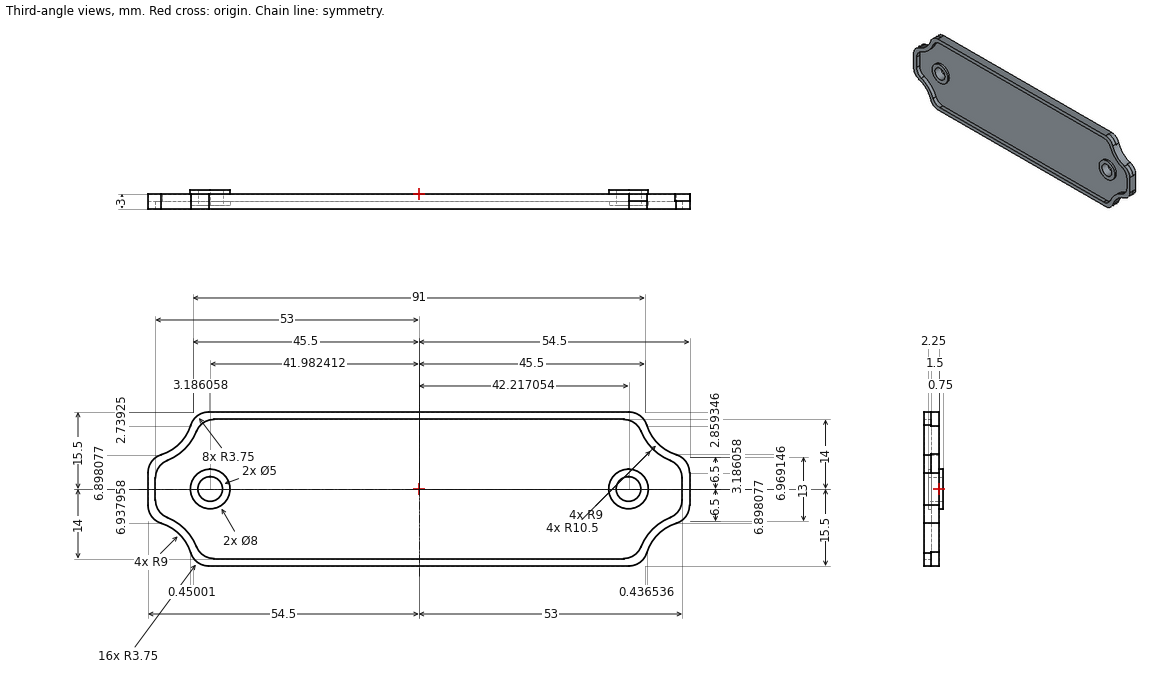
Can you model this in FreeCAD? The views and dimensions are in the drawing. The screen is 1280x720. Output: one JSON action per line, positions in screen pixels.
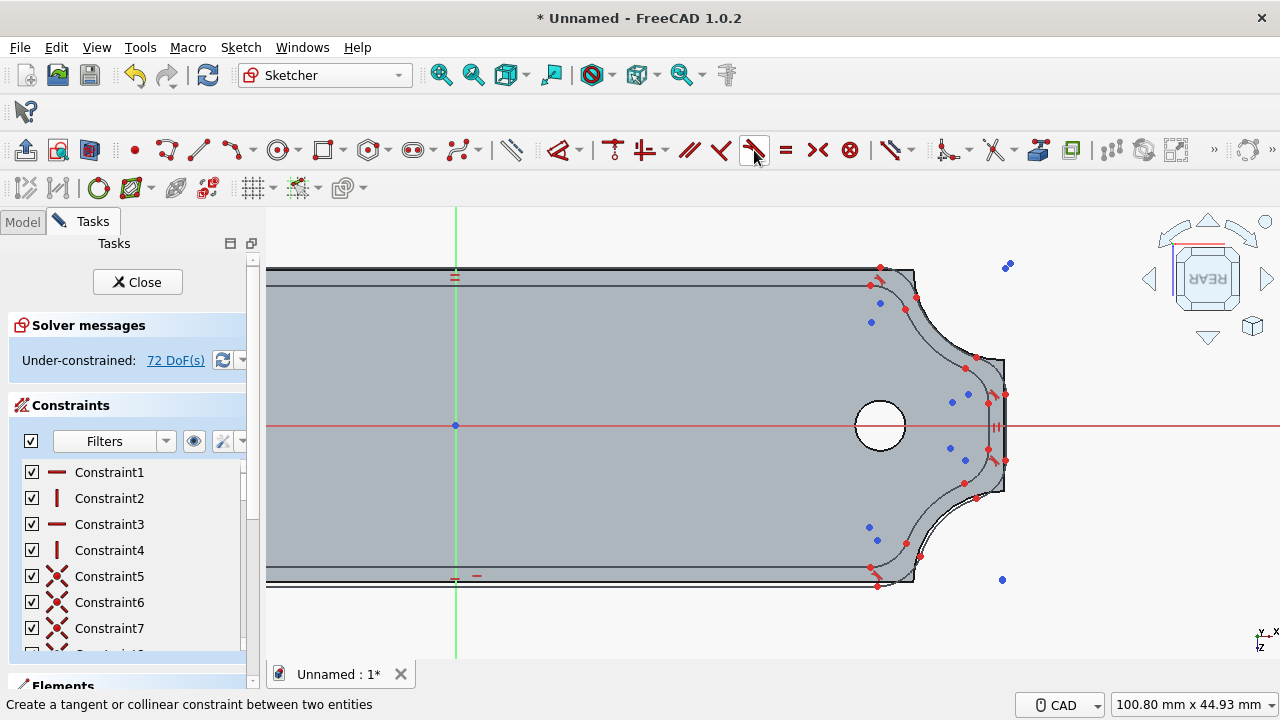
{"action": "scroll", "coordinate": [1007, 442], "scroll_direction": "down", "scroll_amount": 3}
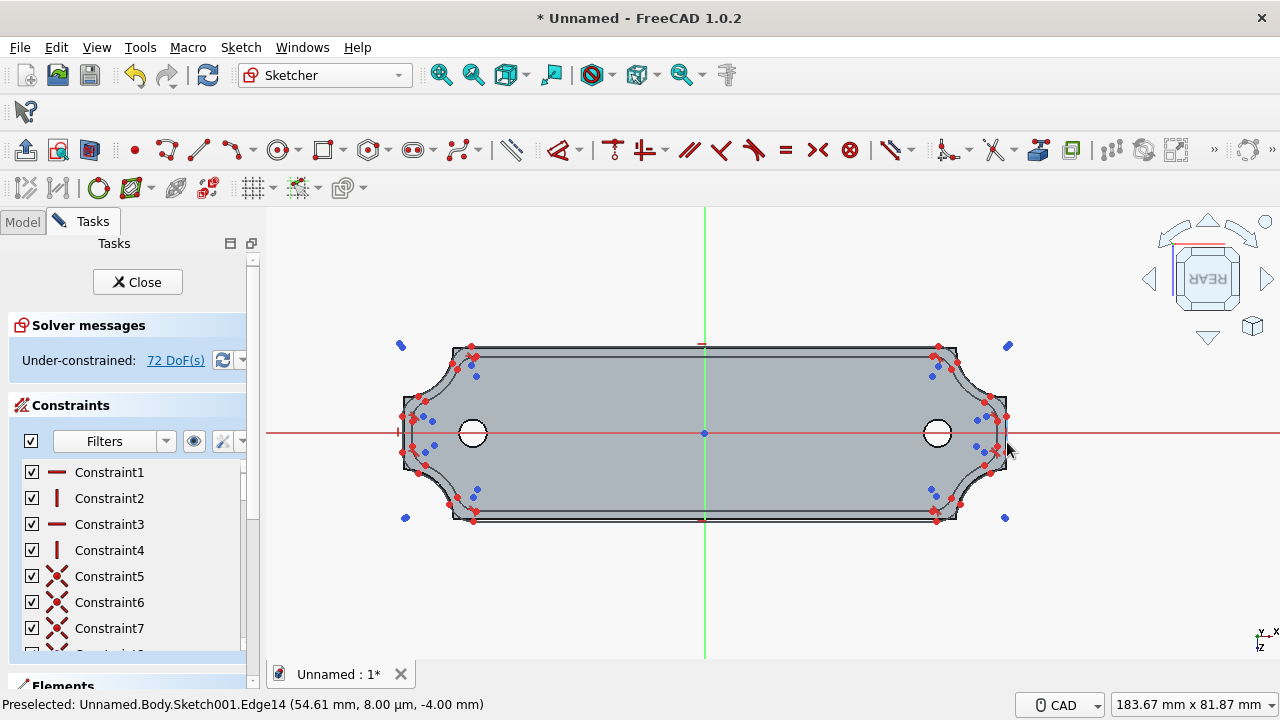
{"action": "scroll", "coordinate": [463, 348], "scroll_direction": "up", "scroll_amount": 3}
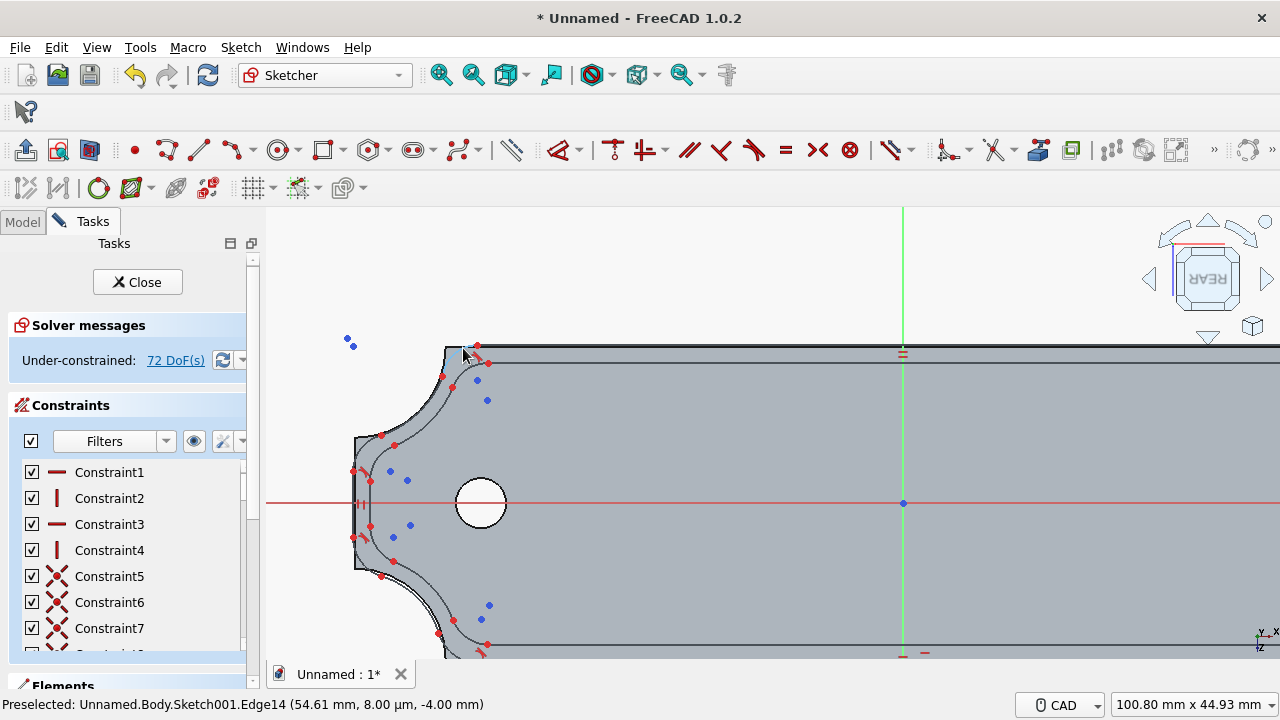
{"action": "left_click", "coordinate": [463, 348]}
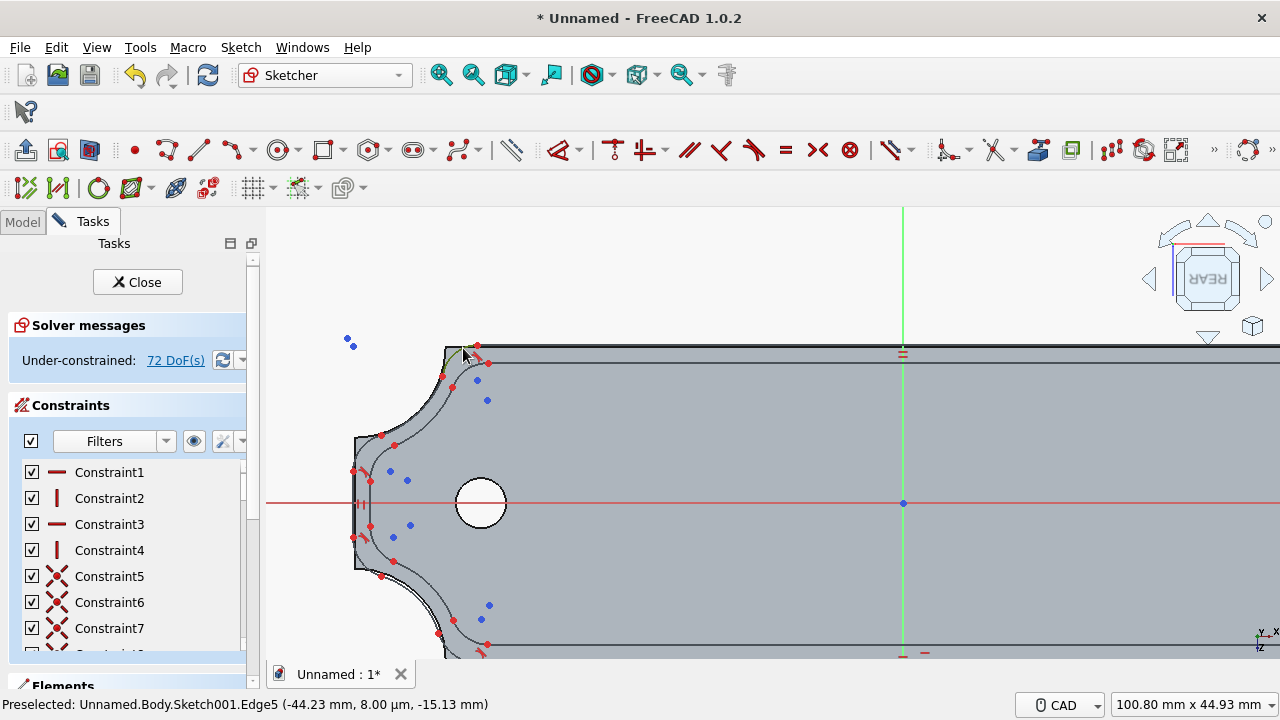
{"action": "left_click", "coordinate": [405, 423]}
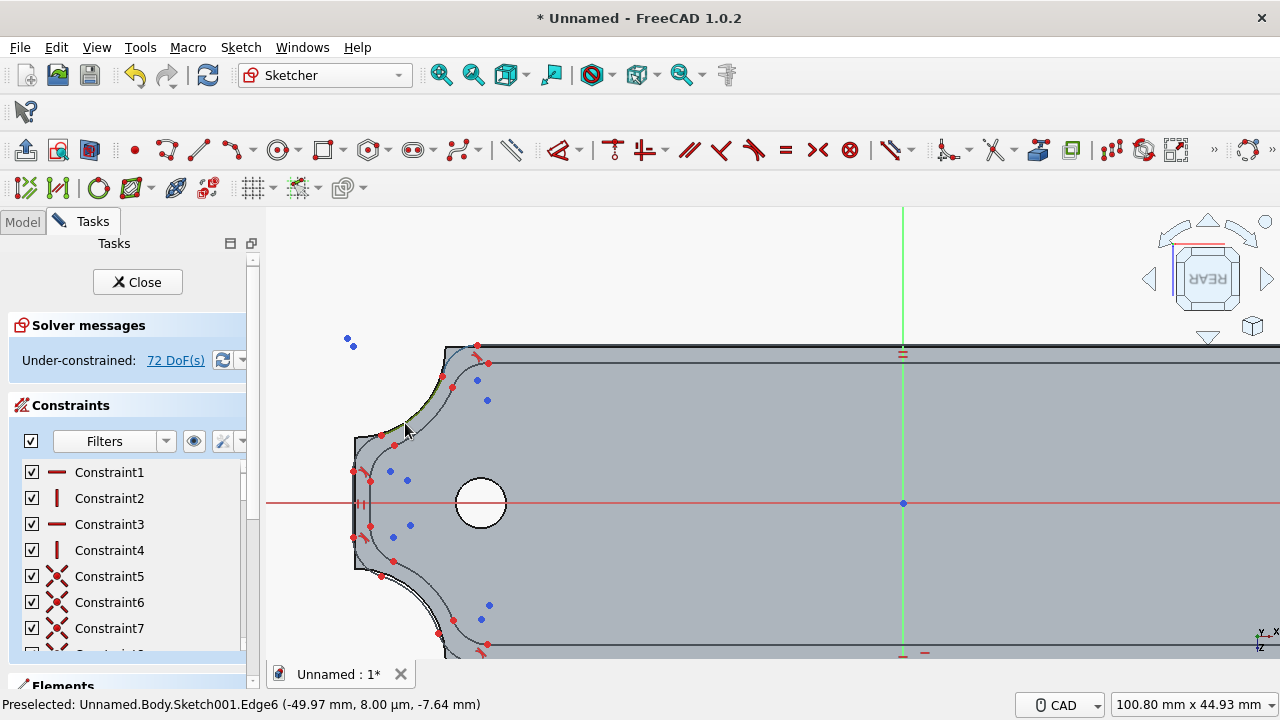
{"action": "left_click", "coordinate": [754, 150]}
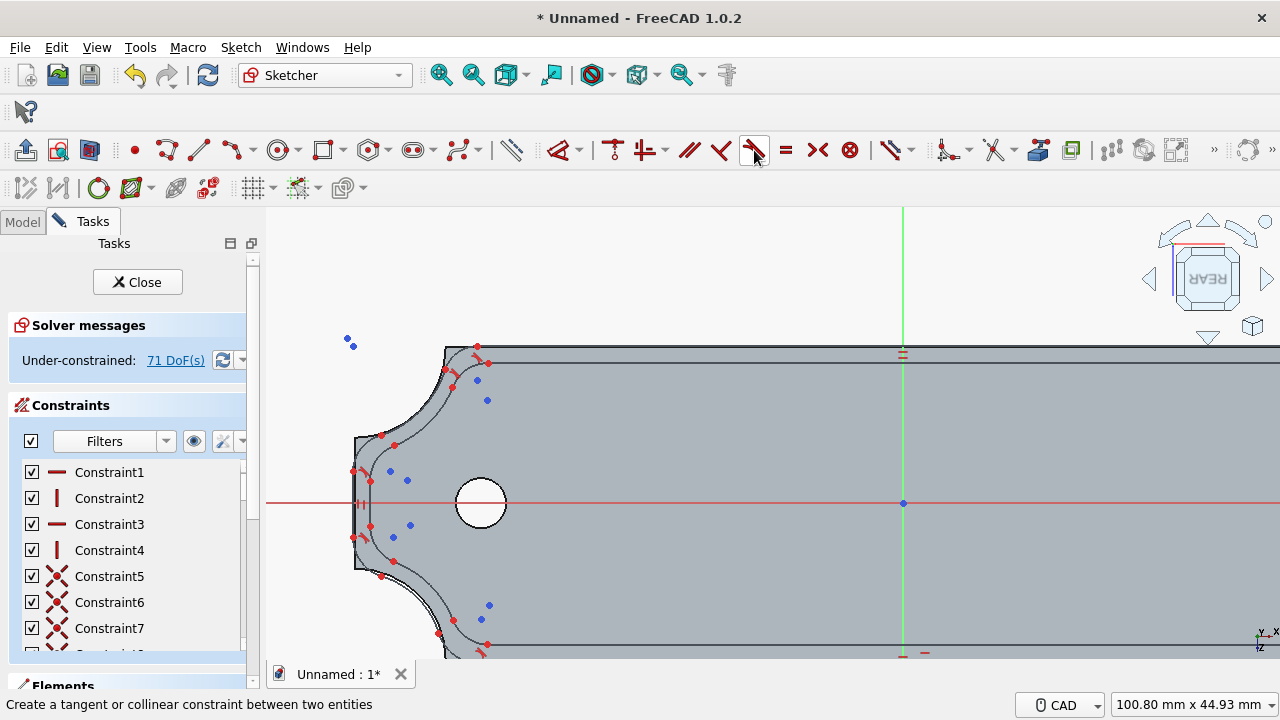
{"action": "left_click", "coordinate": [407, 422]}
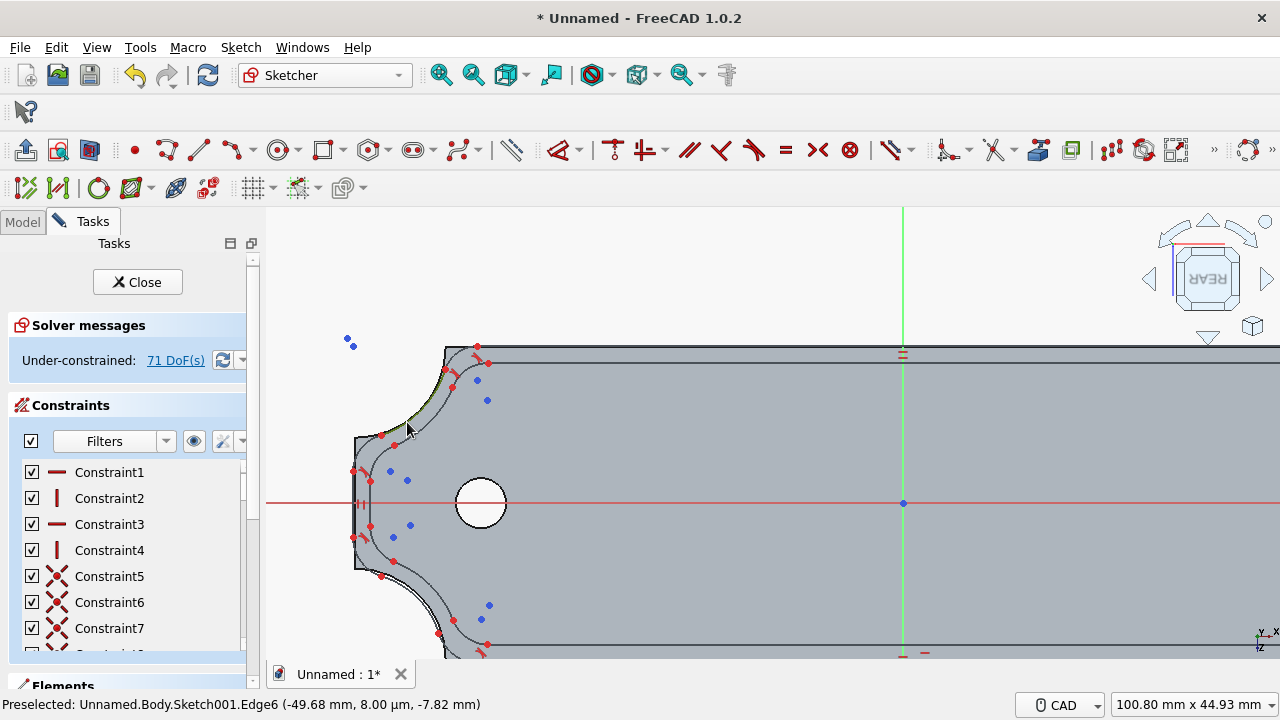
{"action": "left_click", "coordinate": [368, 442]}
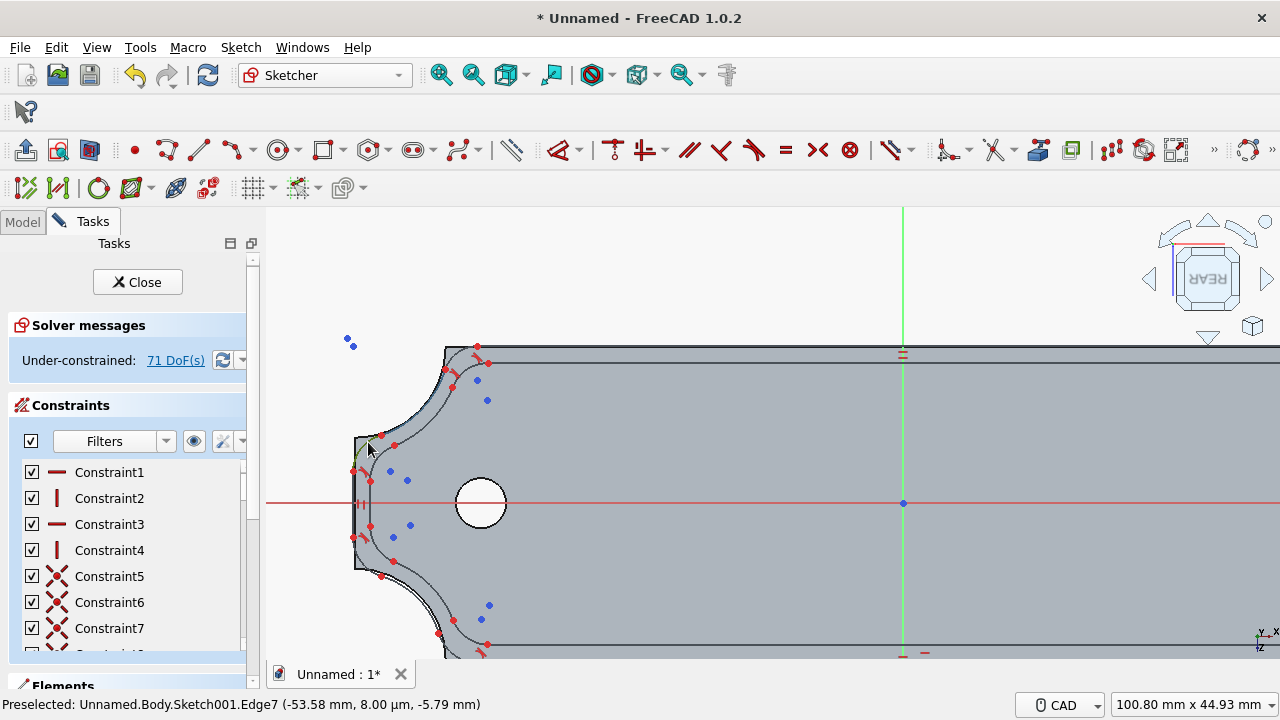
{"action": "left_click", "coordinate": [754, 150]}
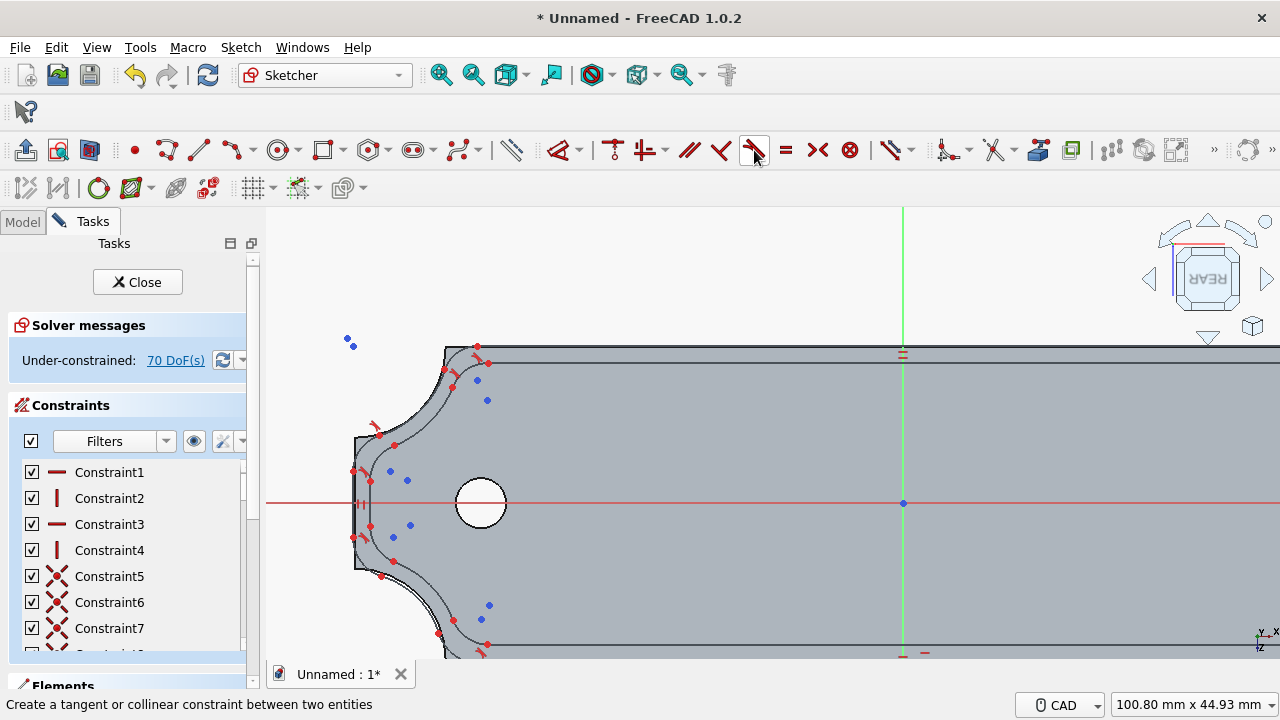
{"action": "left_click", "coordinate": [356, 553]}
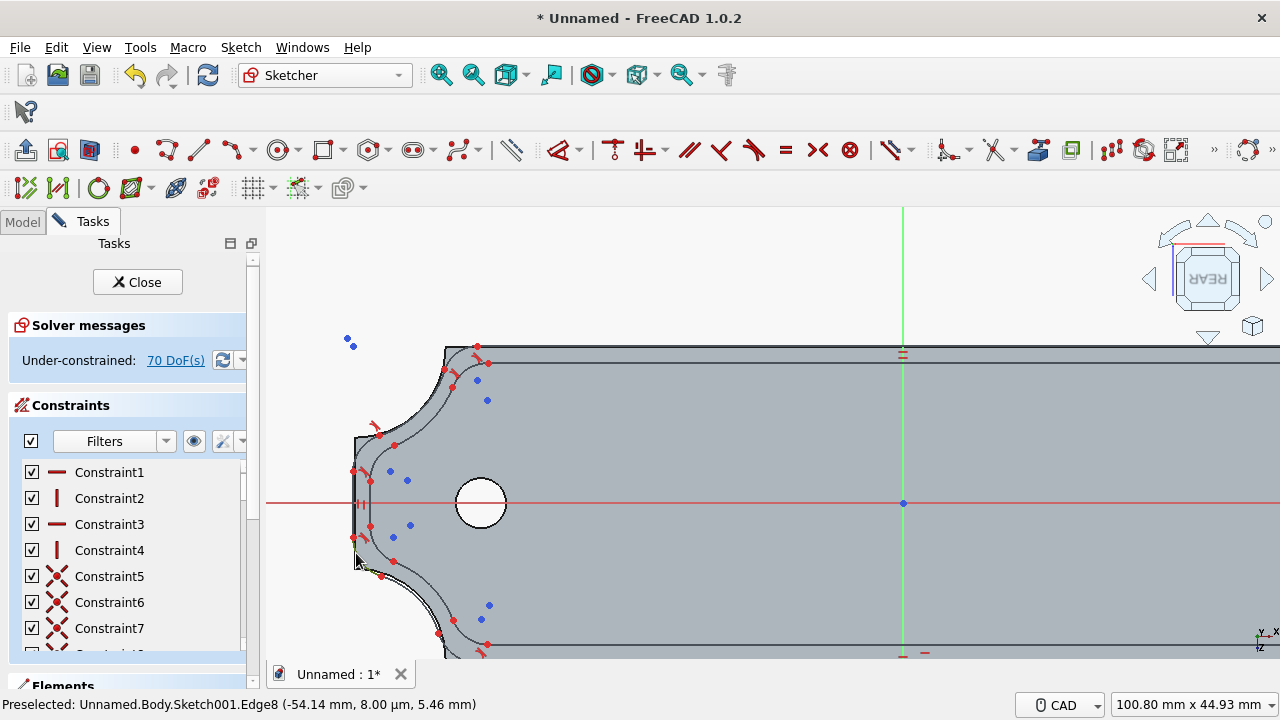
{"action": "left_click", "coordinate": [428, 611]}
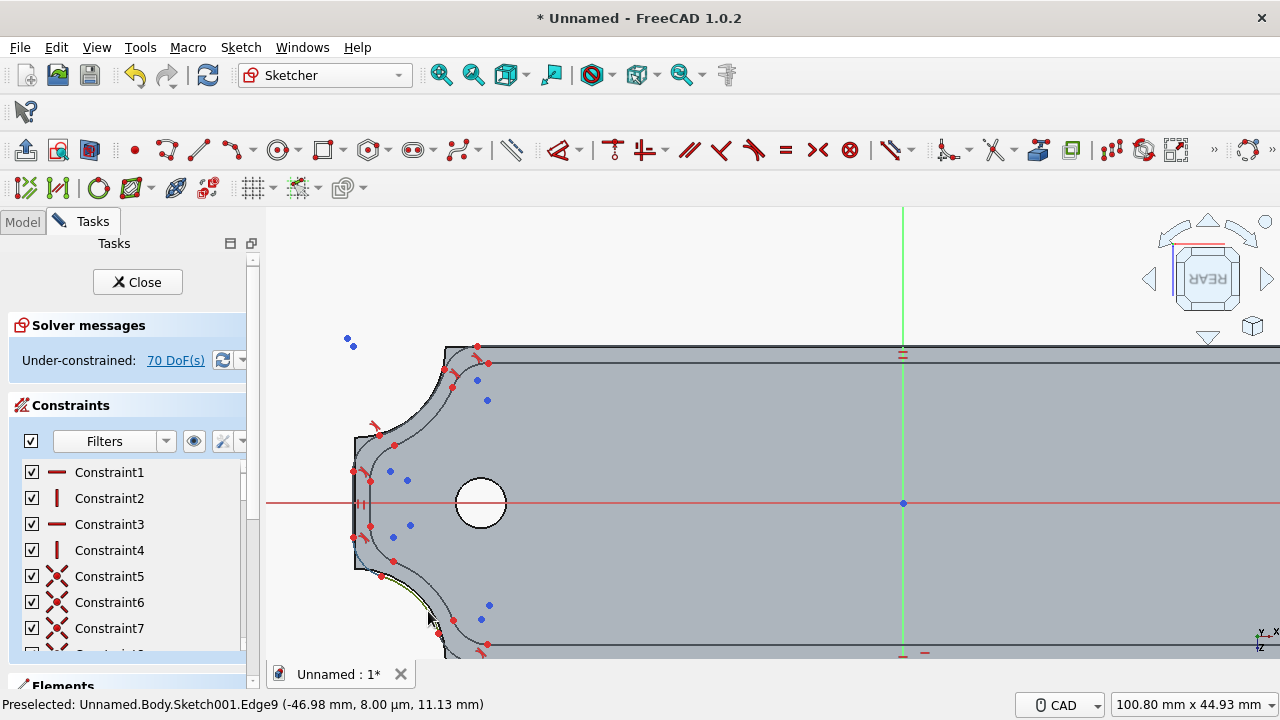
{"action": "left_click", "coordinate": [754, 150]}